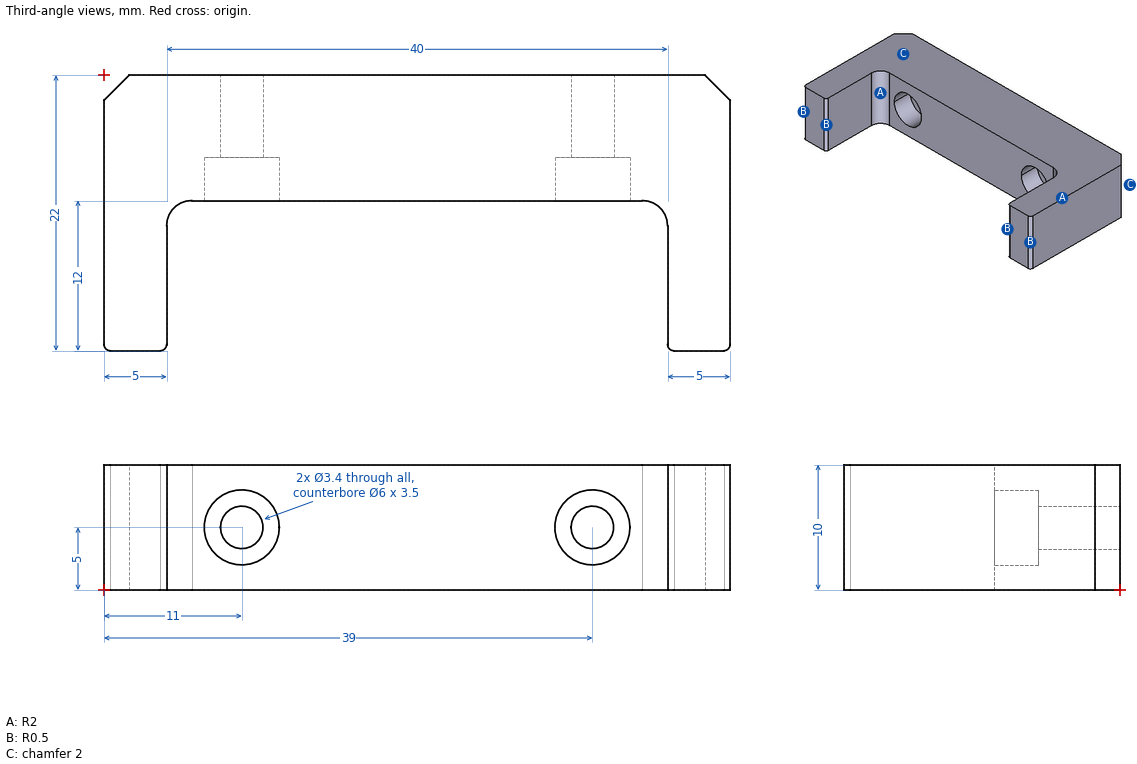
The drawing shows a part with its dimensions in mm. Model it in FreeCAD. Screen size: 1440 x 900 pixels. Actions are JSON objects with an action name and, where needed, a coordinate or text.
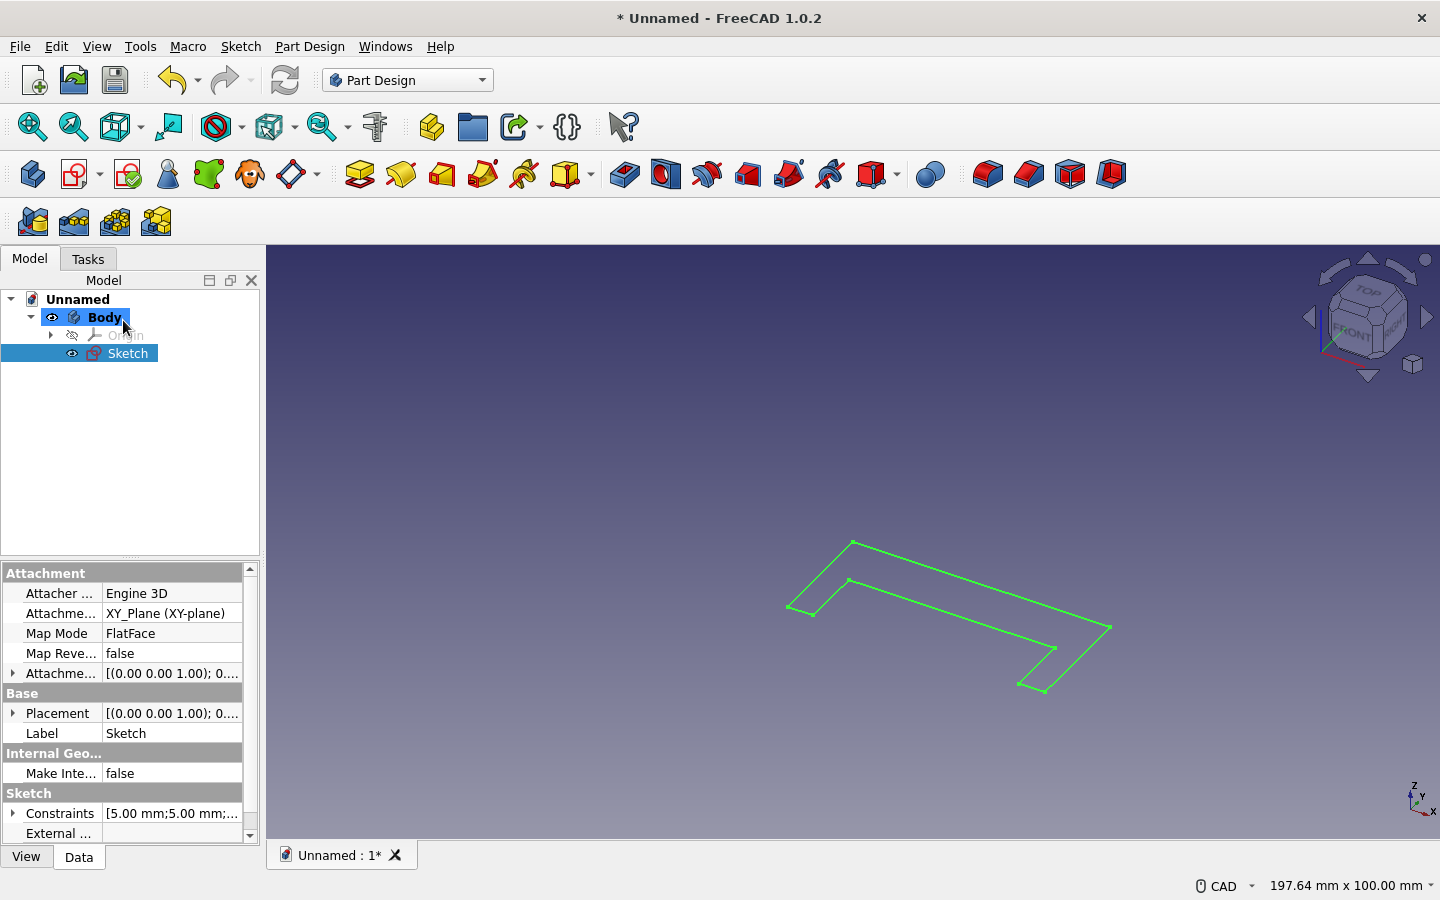
{"action": "left_click", "coordinate": [360, 174]}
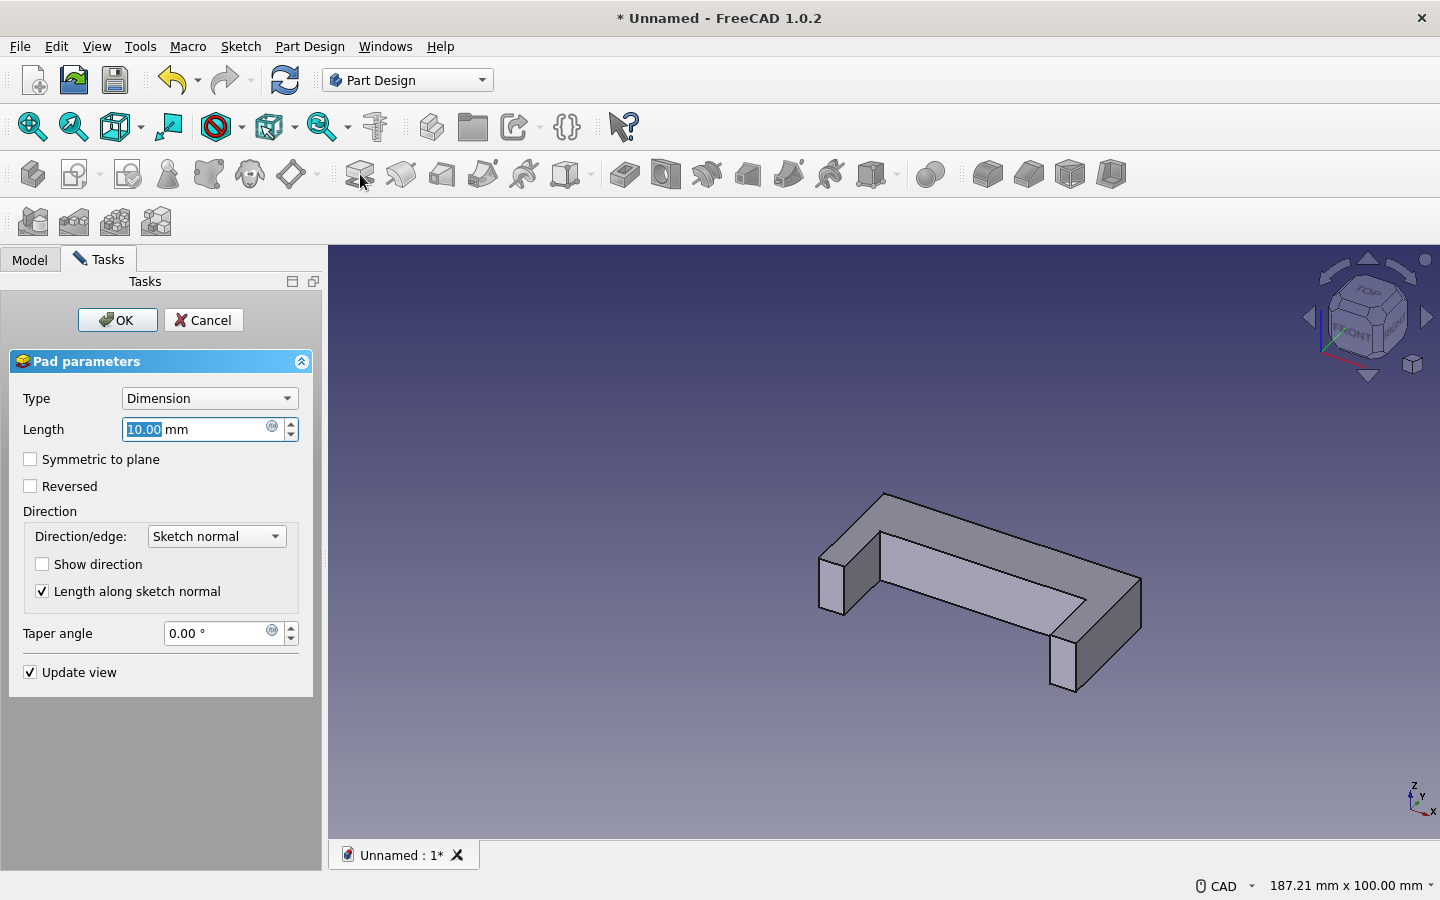
{"action": "type", "text": "10"}
{"action": "key", "text": "Tab"}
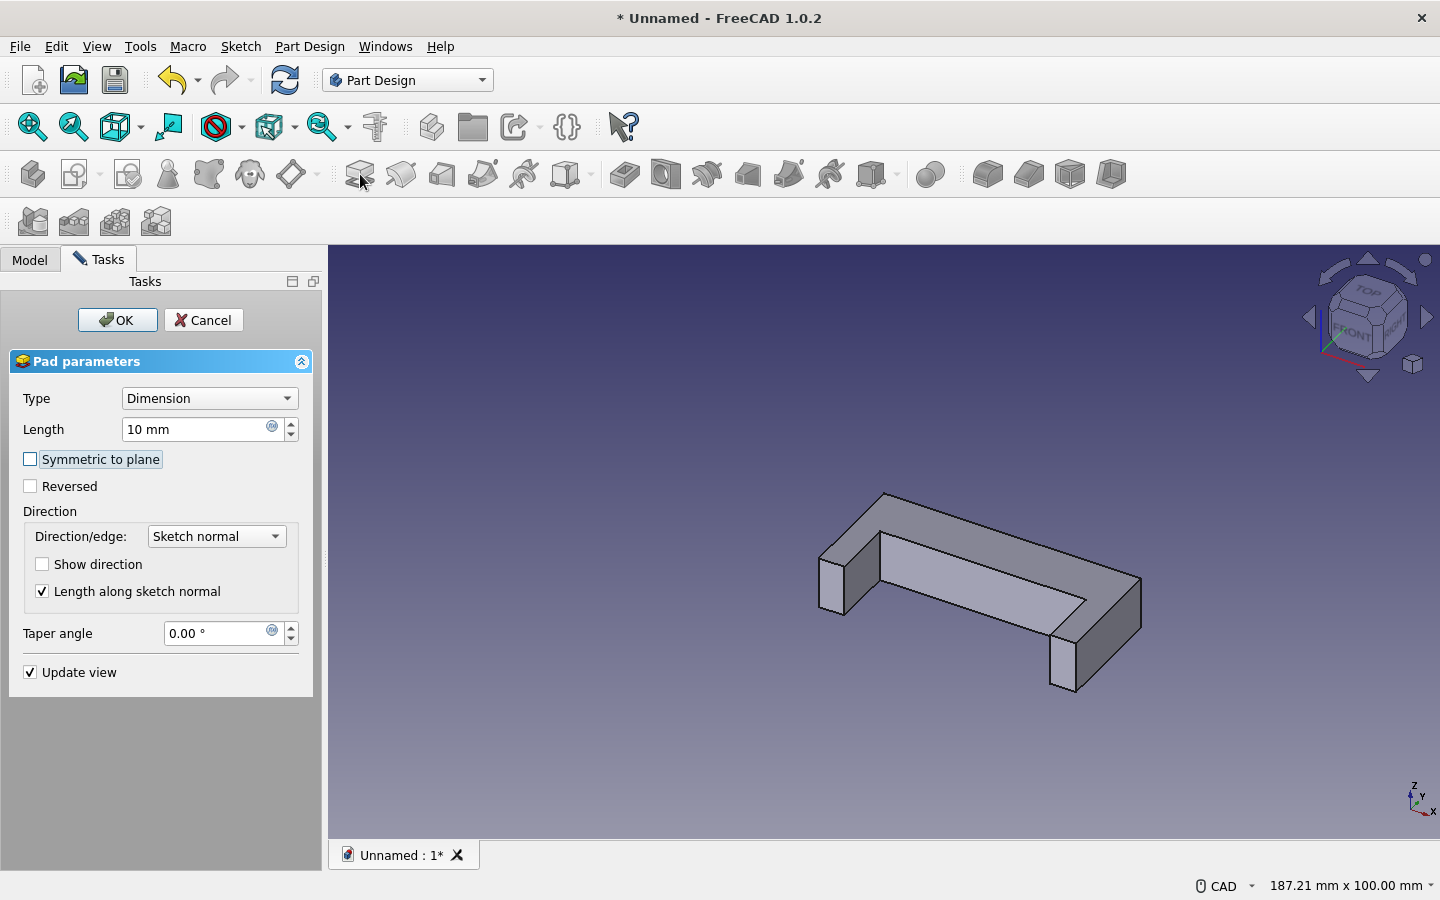
{"action": "left_click", "coordinate": [118, 320]}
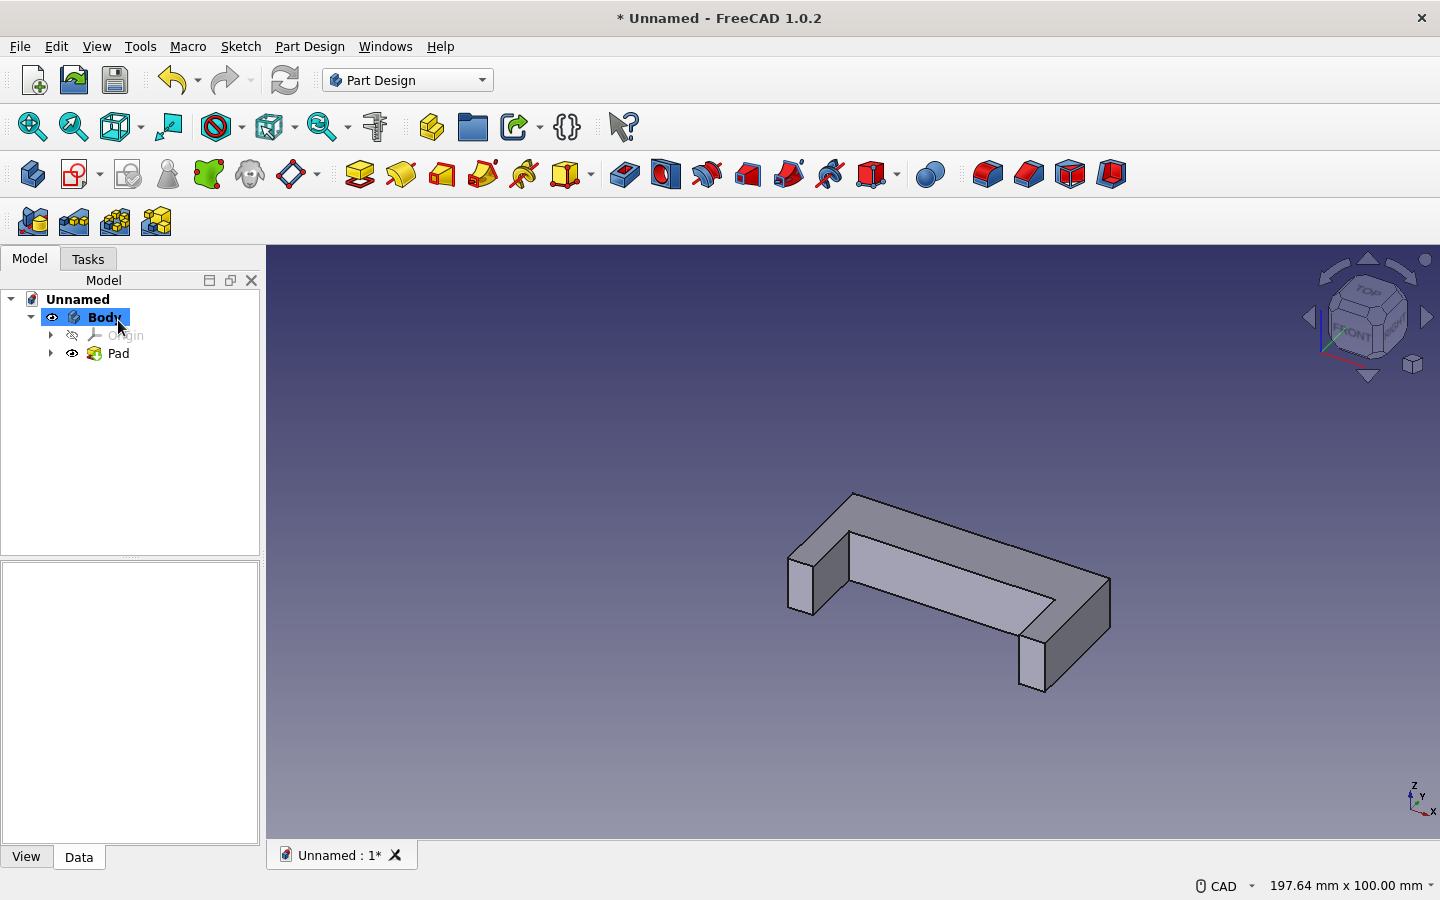
{"action": "left_click", "coordinate": [33, 128]}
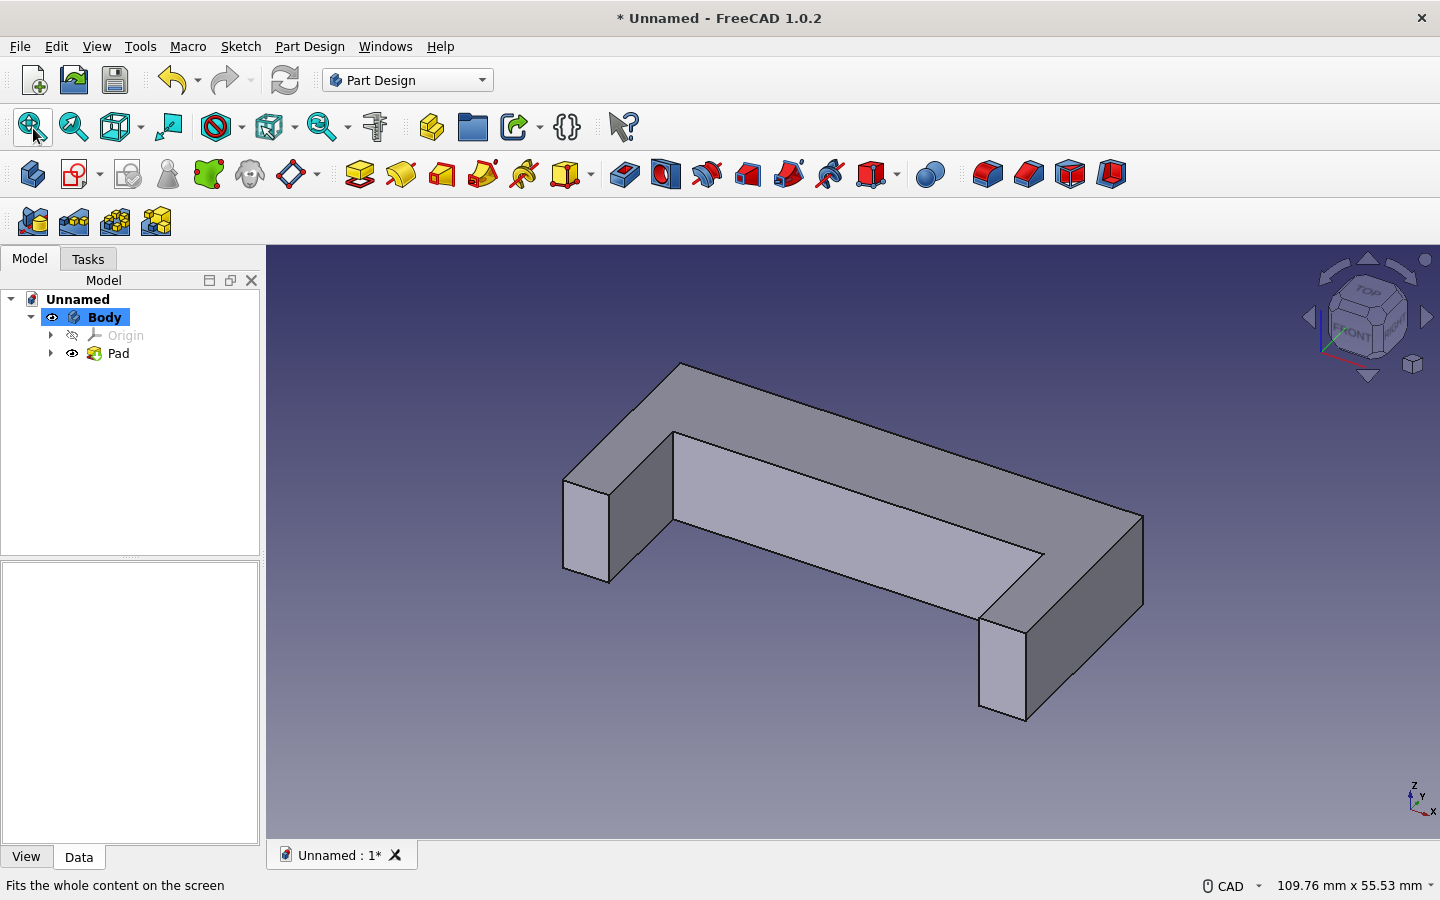
{"action": "left_click", "coordinate": [964, 571]}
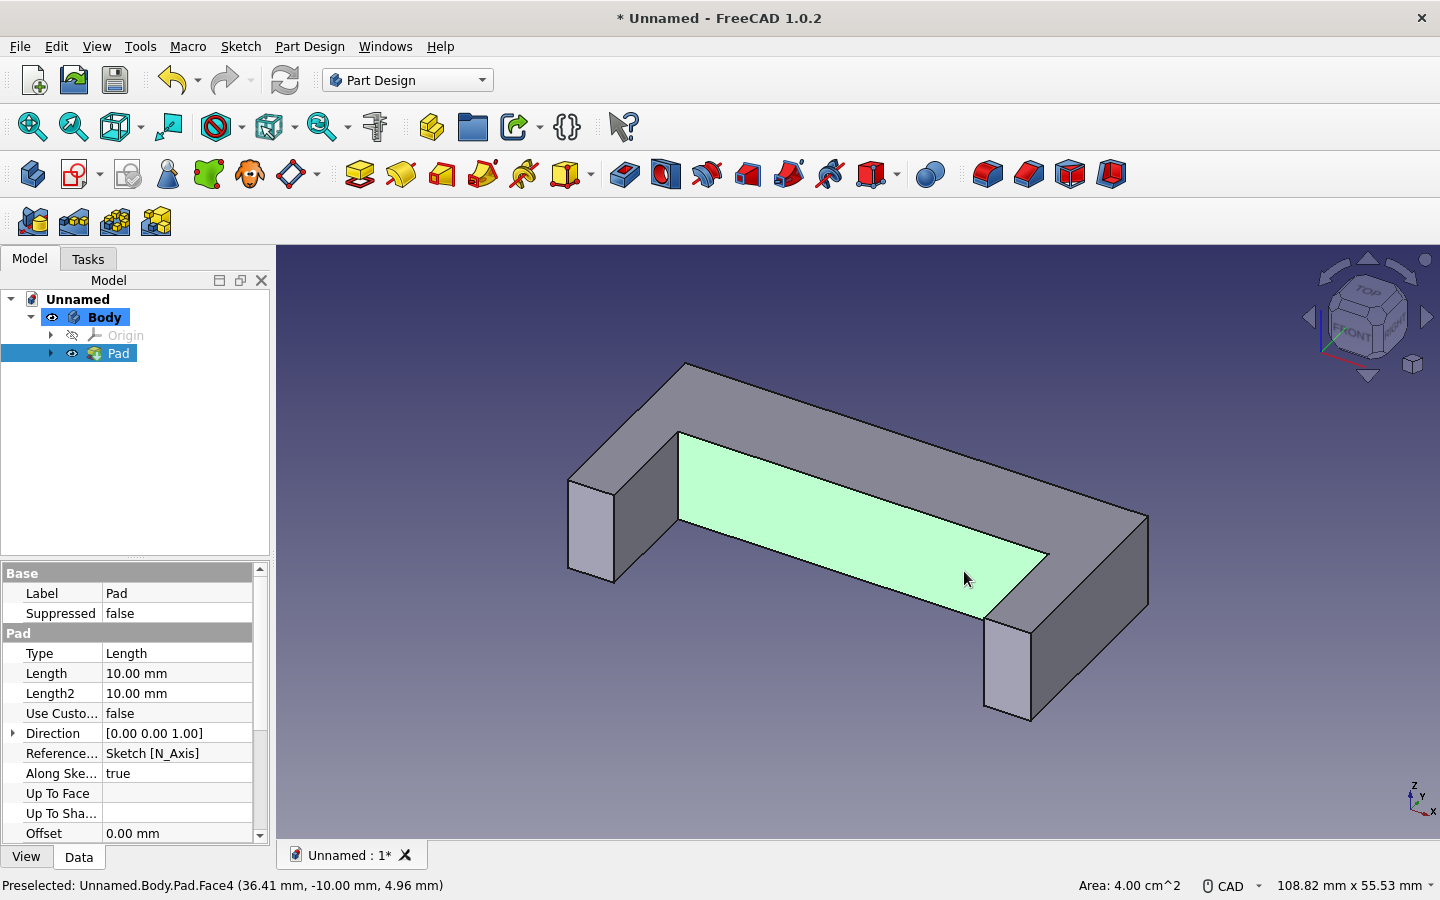
{"action": "left_click", "coordinate": [74, 174]}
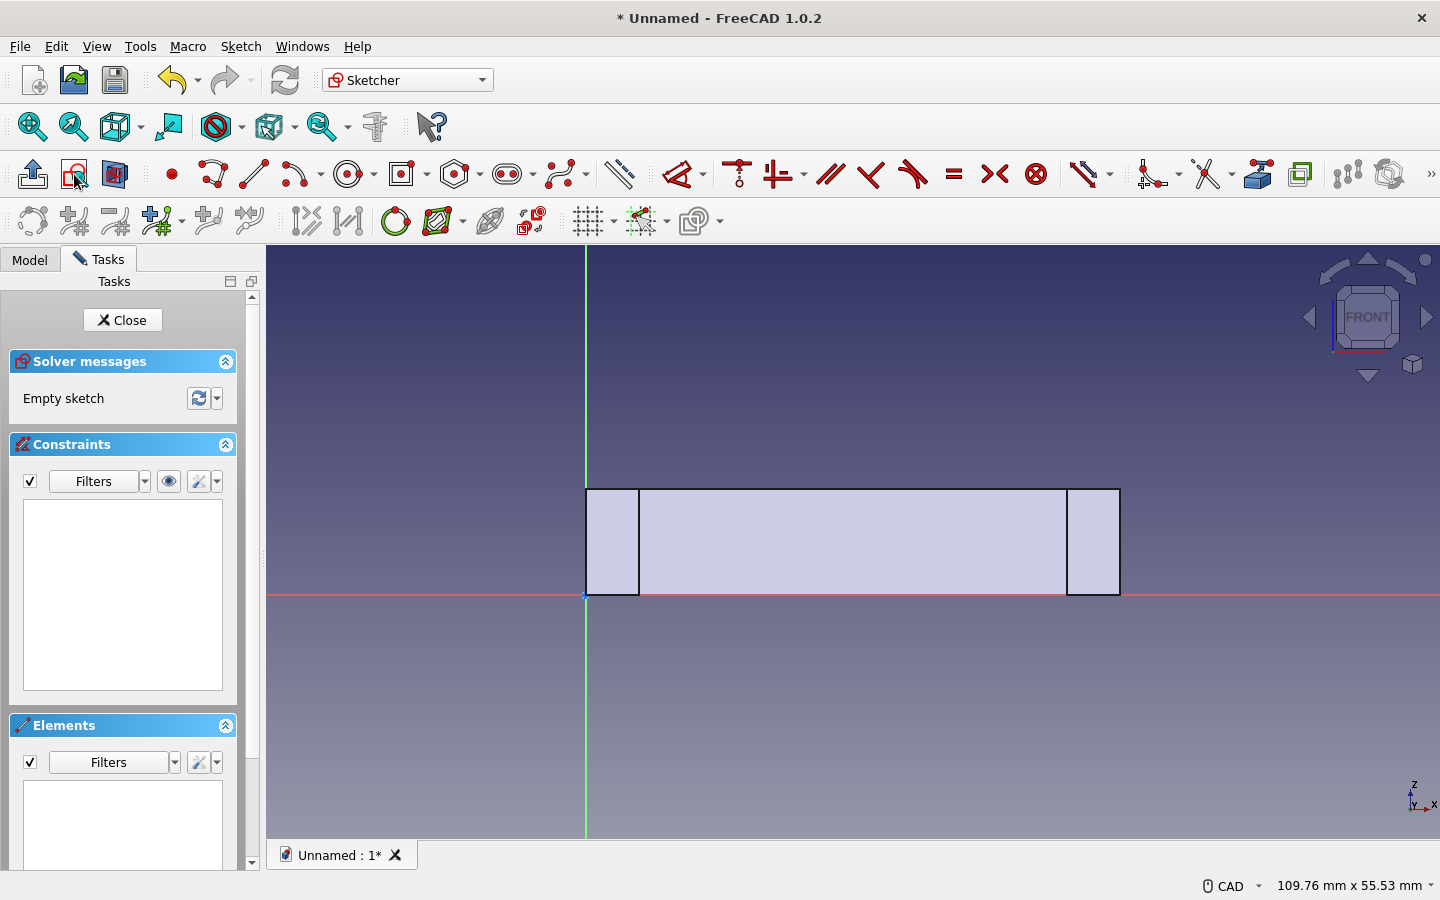
{"action": "left_click", "coordinate": [115, 174]}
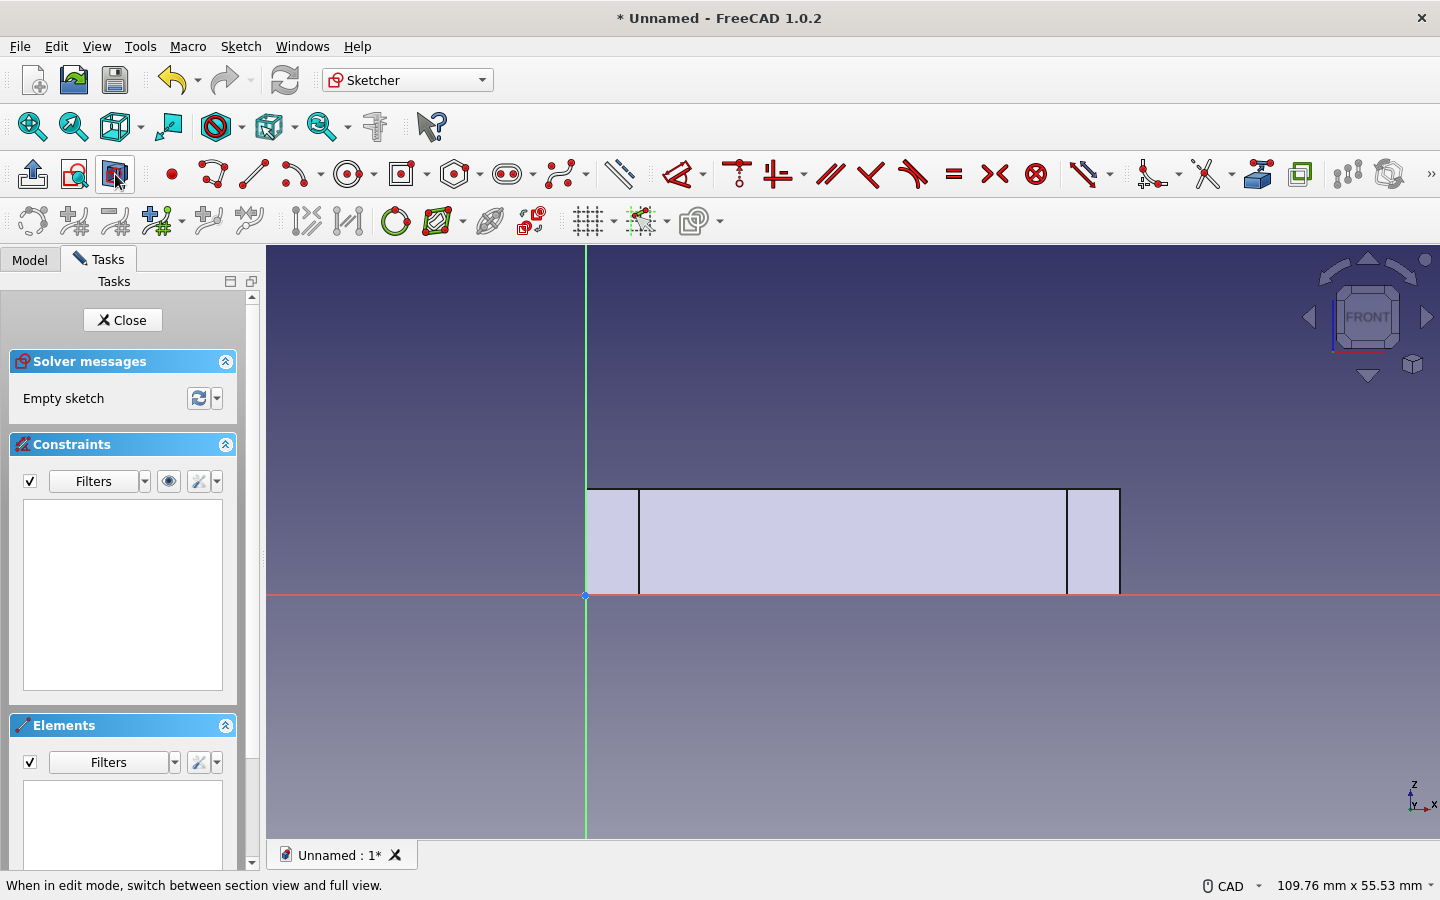
{"action": "scroll", "coordinate": [841, 596], "scroll_direction": "up", "scroll_amount": 2}